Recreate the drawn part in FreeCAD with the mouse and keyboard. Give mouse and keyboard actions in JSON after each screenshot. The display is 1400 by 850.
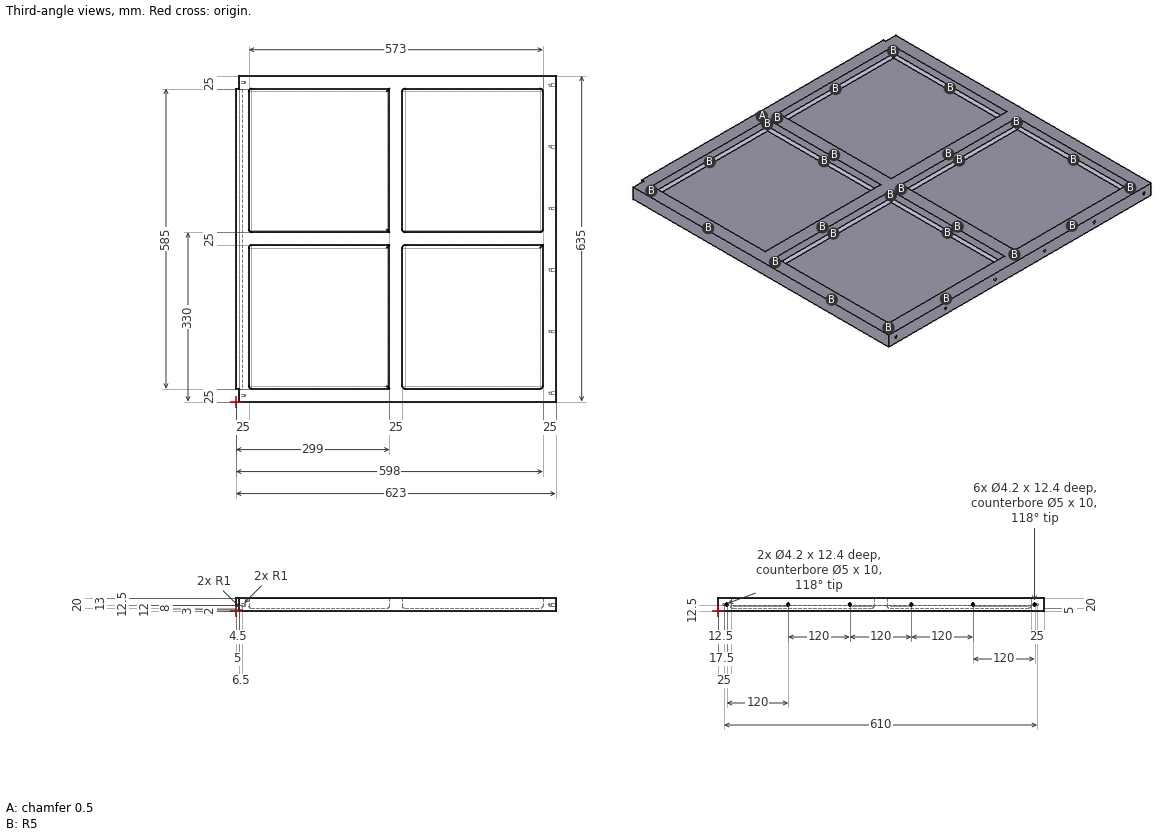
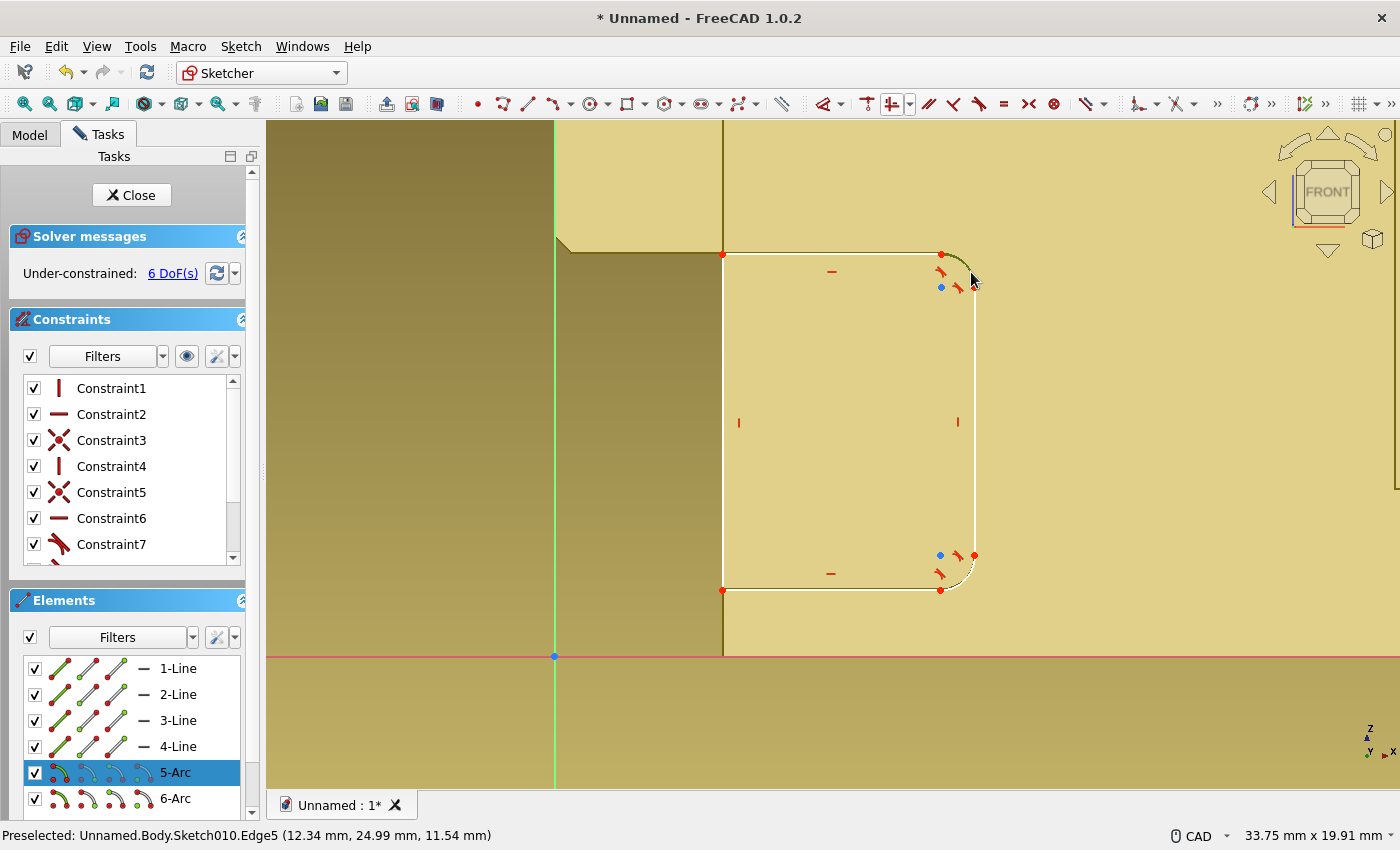
{"action": "left_click", "coordinate": [956, 587]}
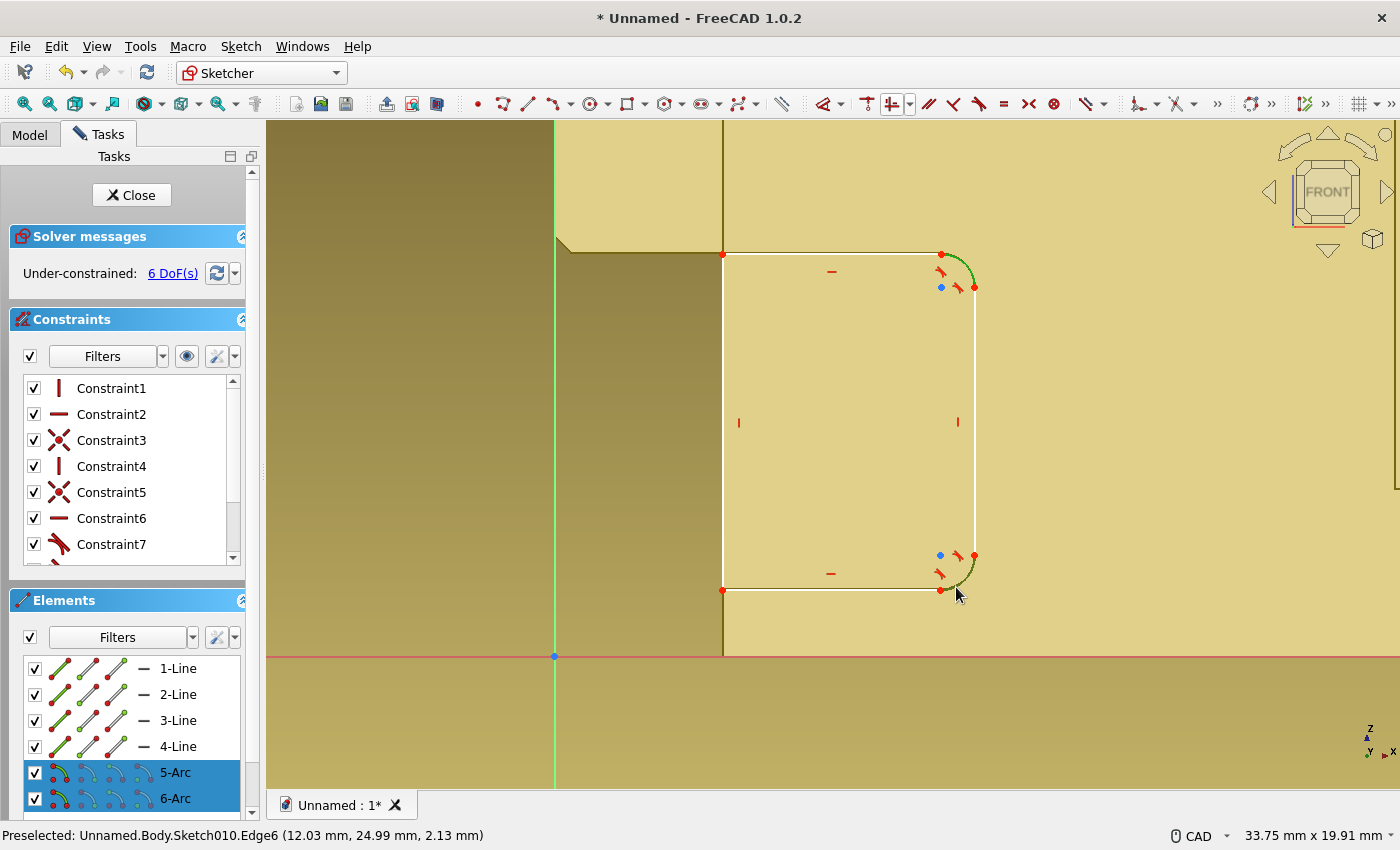
{"action": "left_click", "coordinate": [1004, 104]}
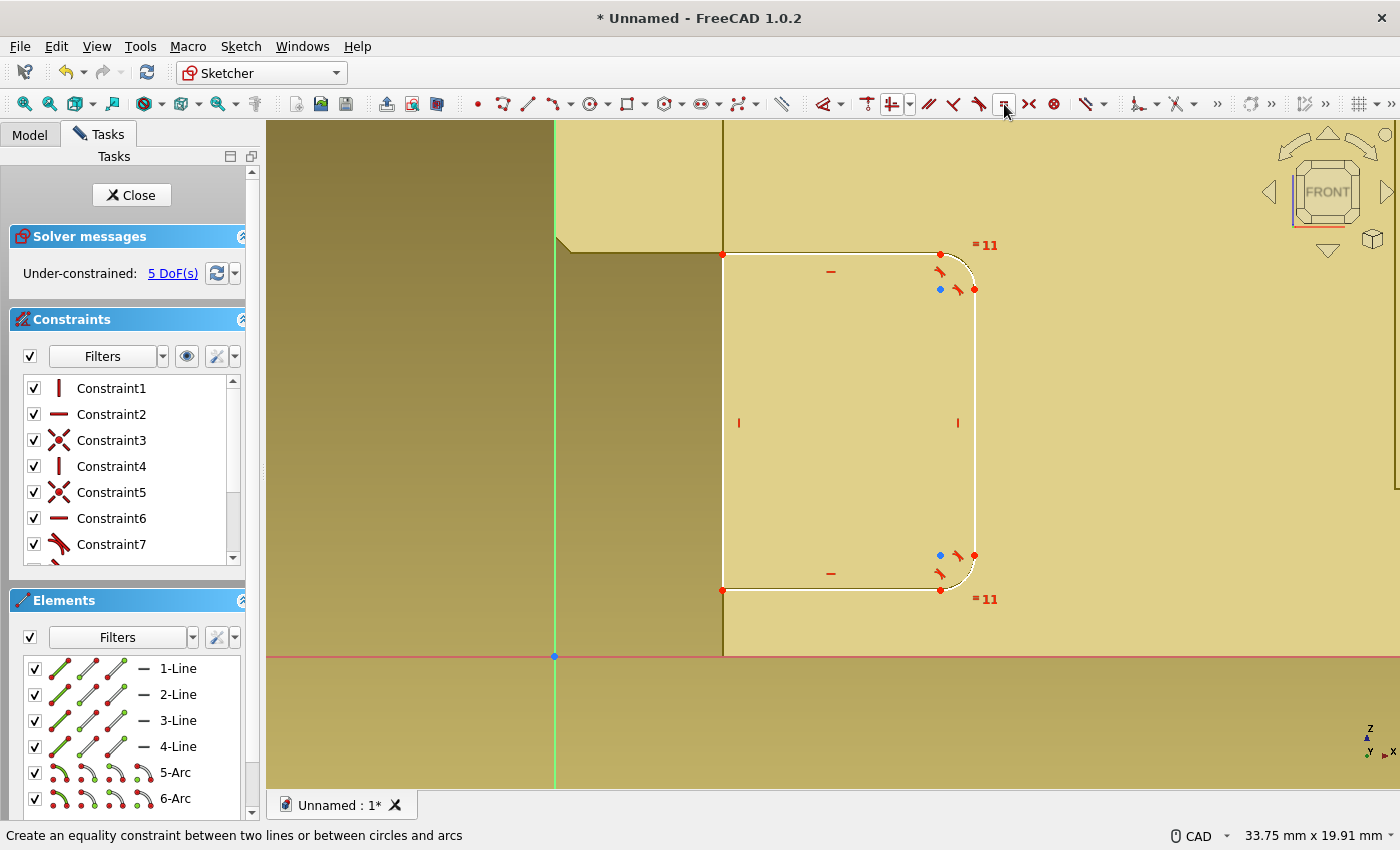
{"action": "key", "text": "d"}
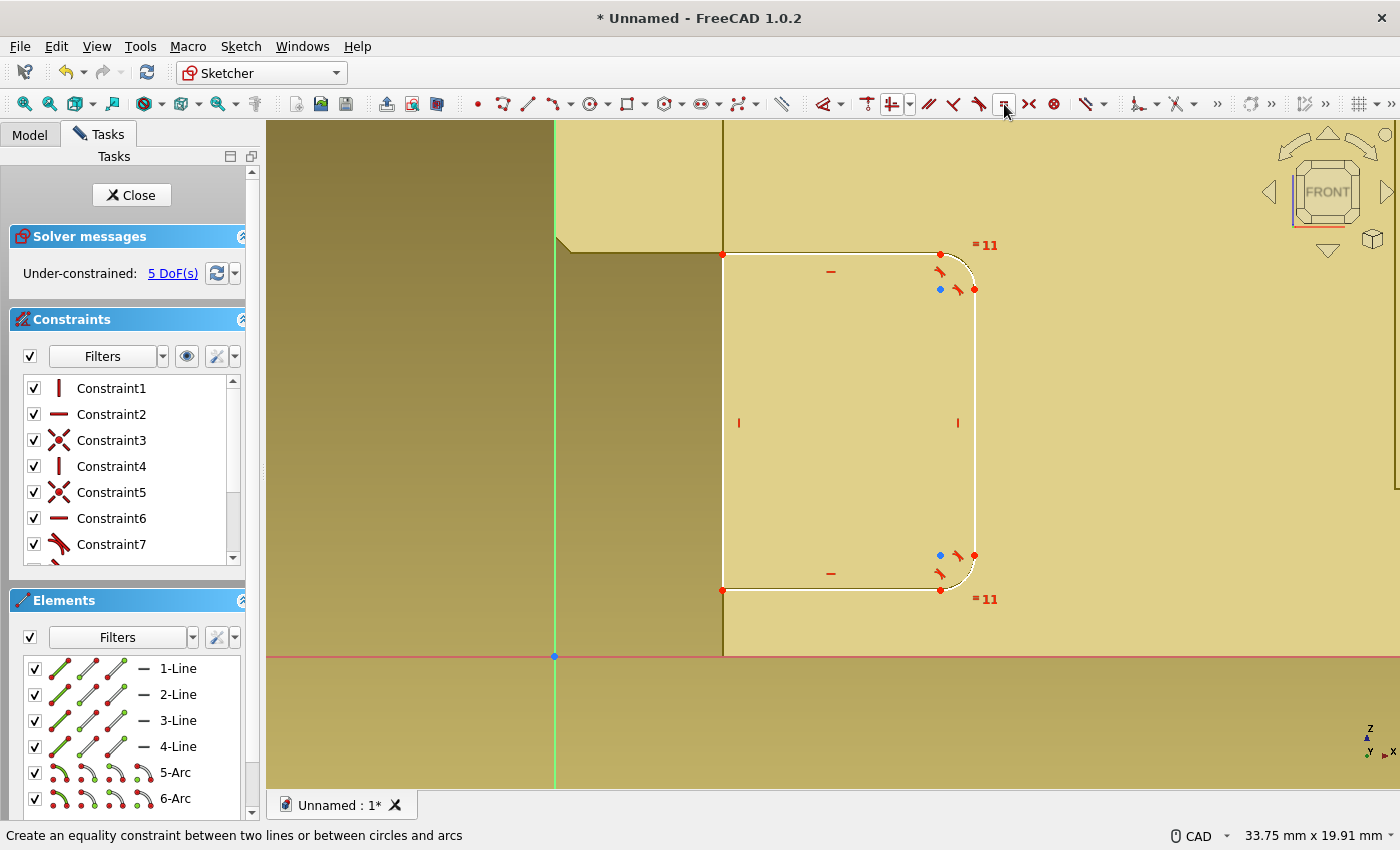
{"action": "left_click", "coordinate": [971, 273]}
{"action": "left_click", "coordinate": [999, 258]}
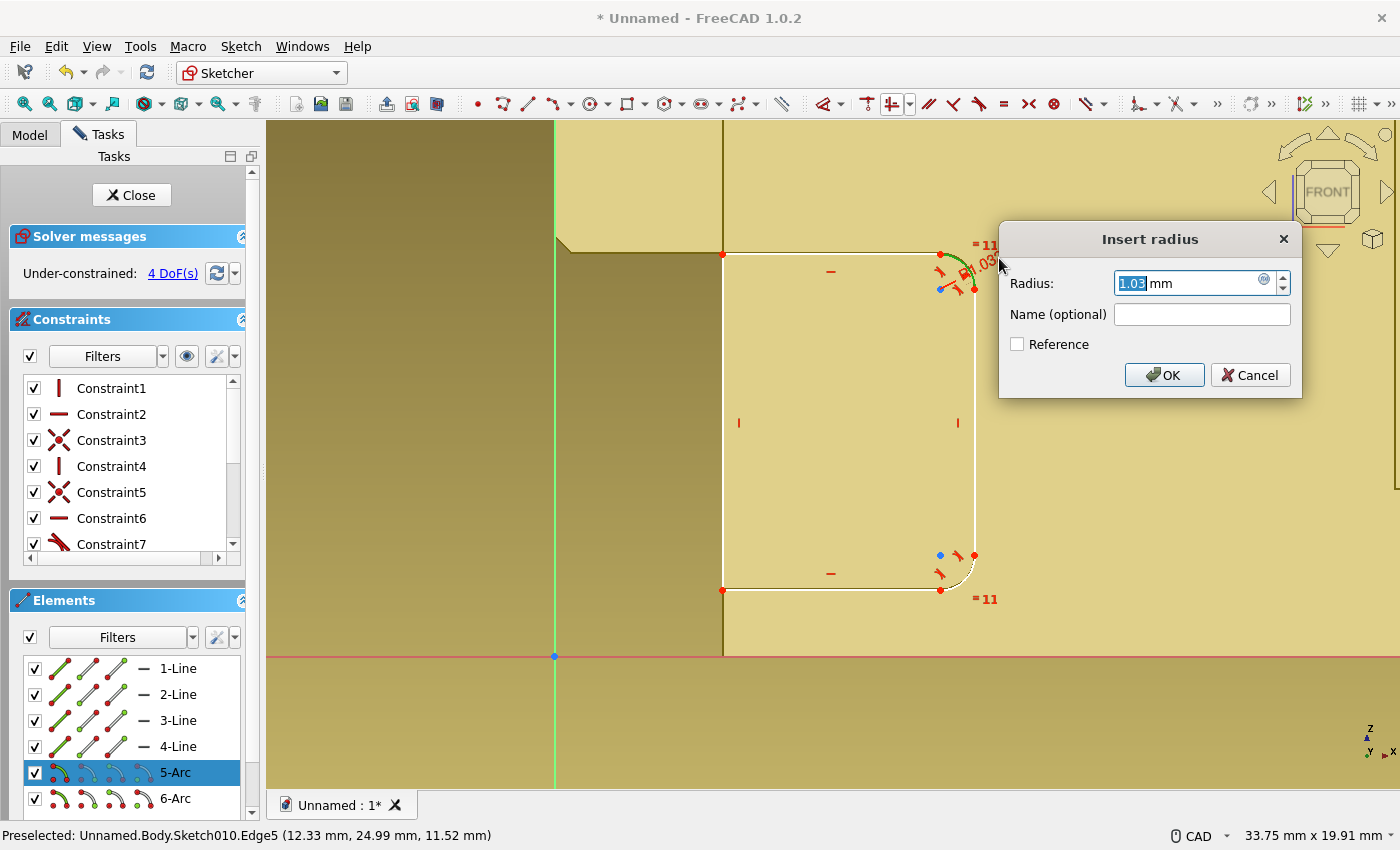
{"action": "type", "text": "1"}
{"action": "key", "text": "Return"}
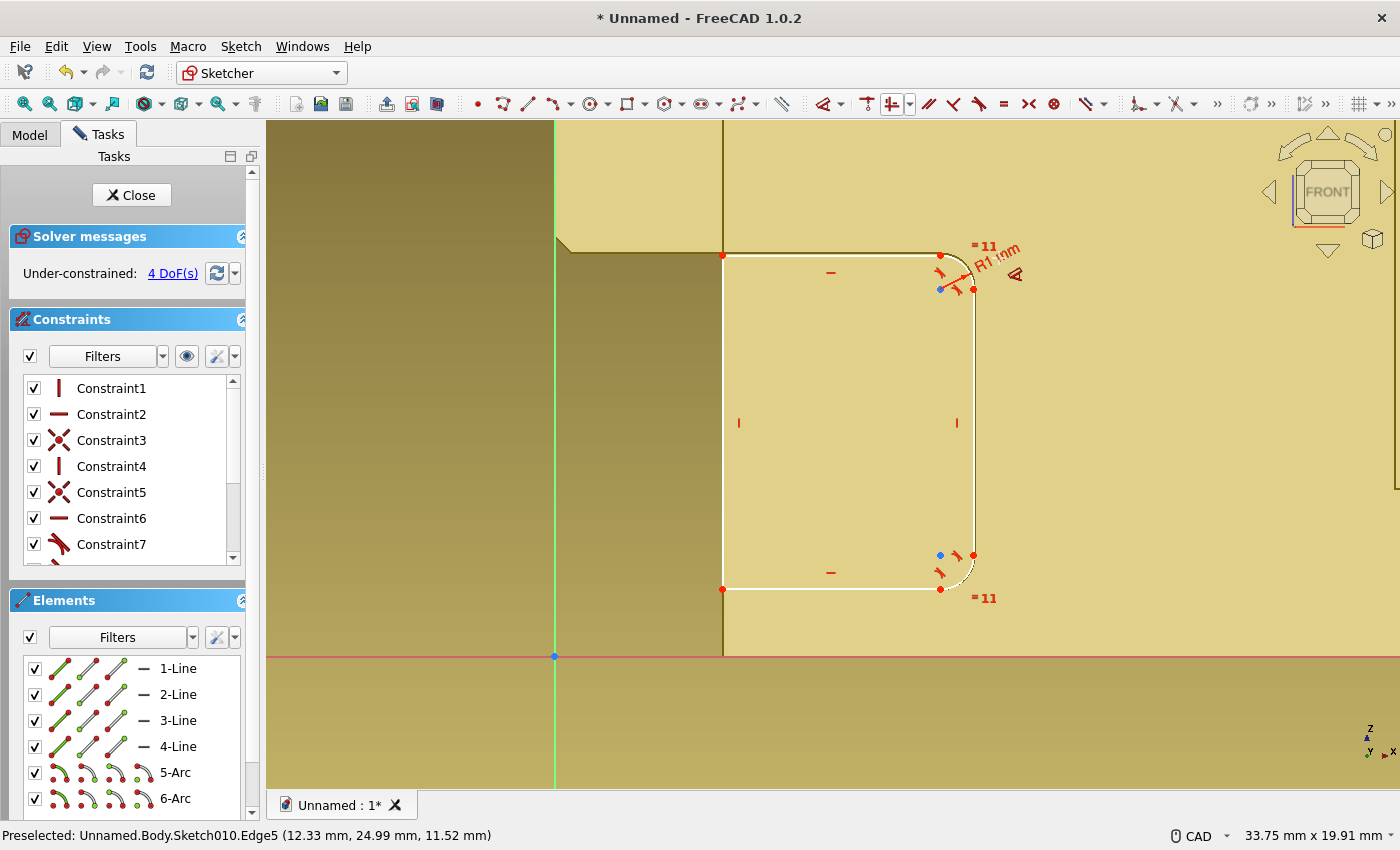
{"action": "left_click", "coordinate": [974, 476]}
{"action": "left_click", "coordinate": [1008, 422]}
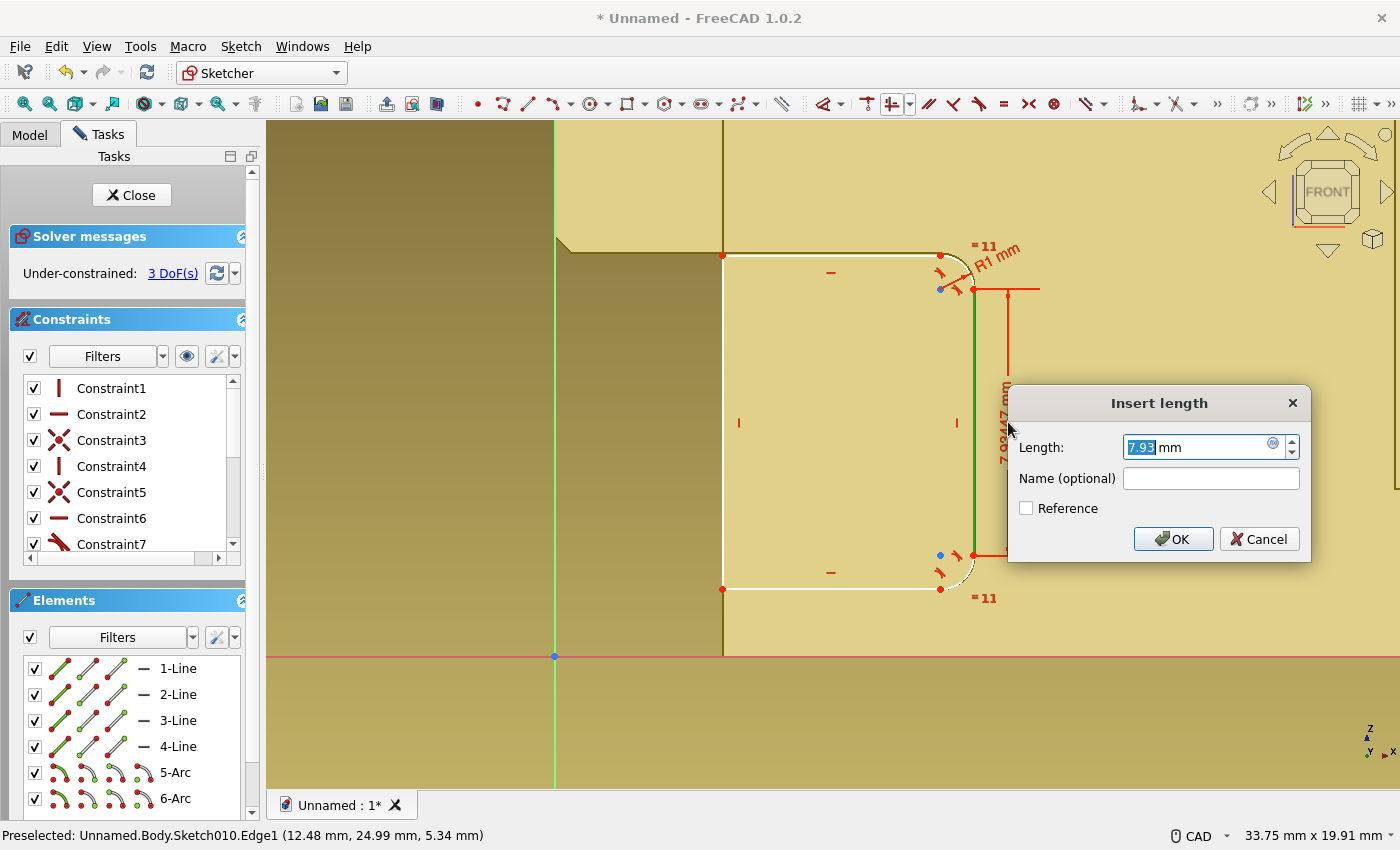
{"action": "type", "text": "8"}
{"action": "key", "text": "Return"}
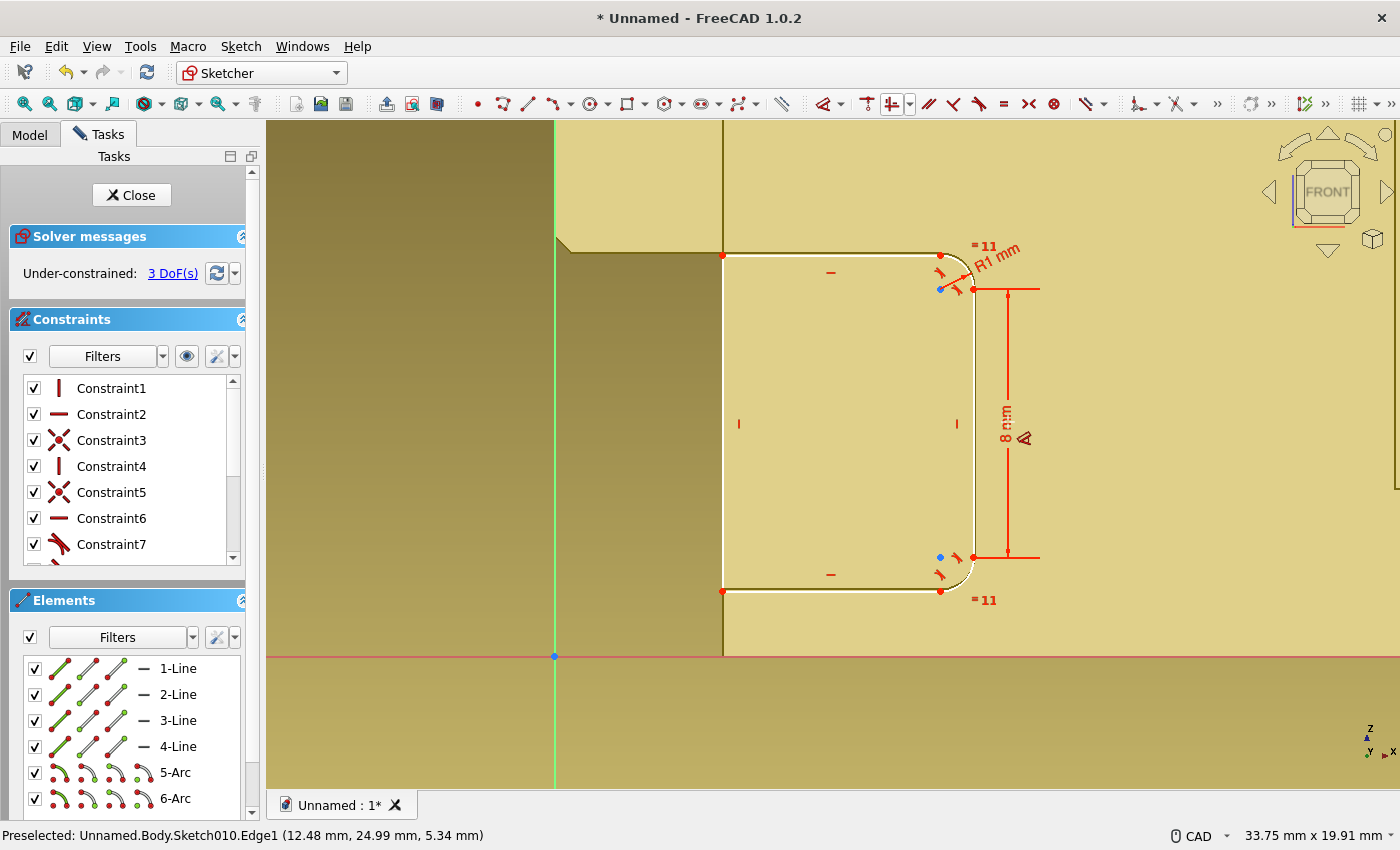
{"action": "left_click", "coordinate": [974, 558]}
{"action": "left_click", "coordinate": [521, 607]}